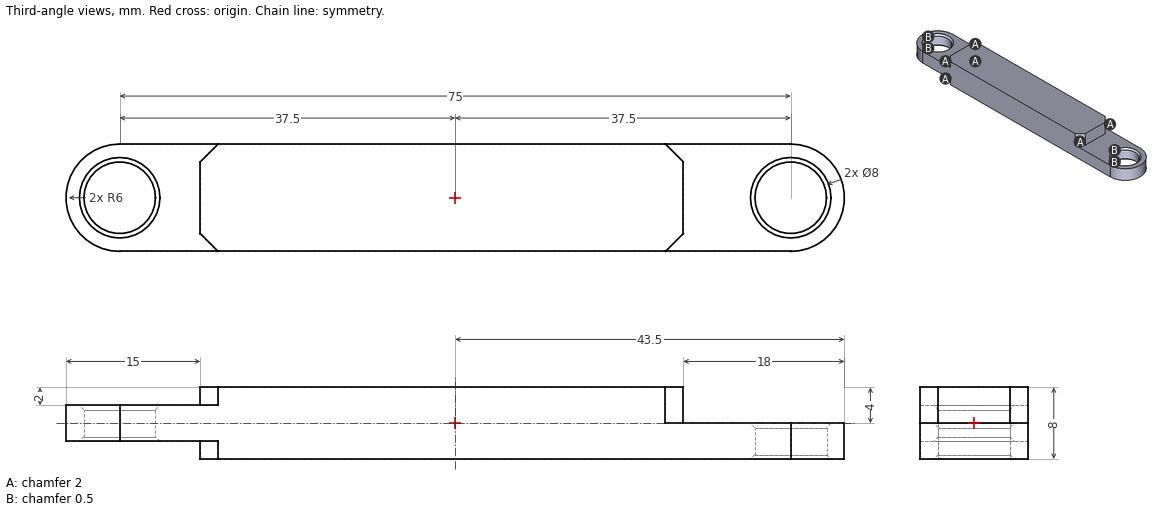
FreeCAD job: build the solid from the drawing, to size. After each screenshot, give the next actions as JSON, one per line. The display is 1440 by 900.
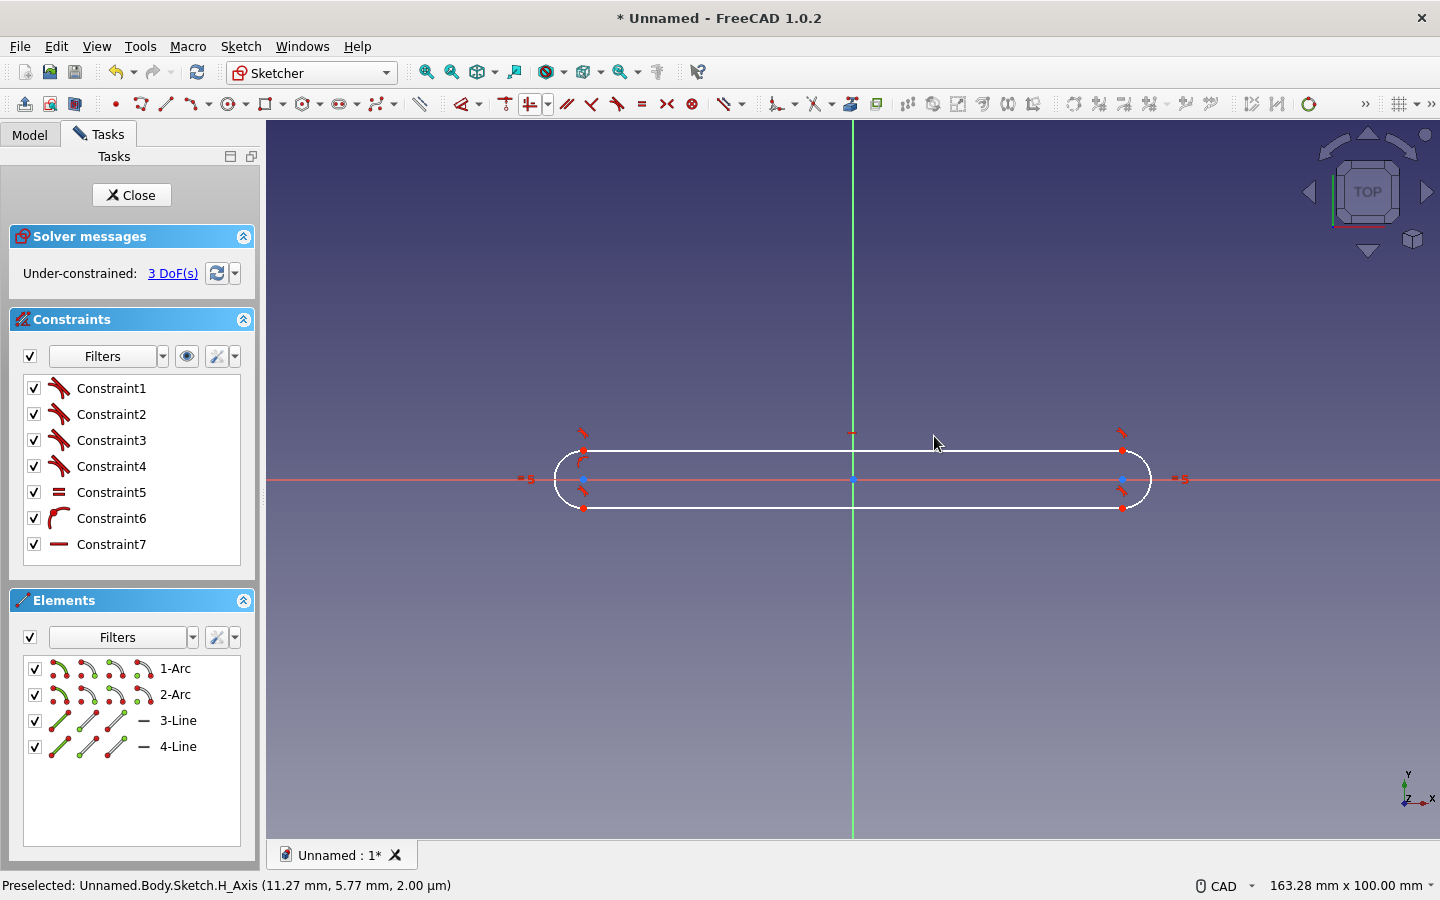
{"action": "left_click", "coordinate": [460, 104]}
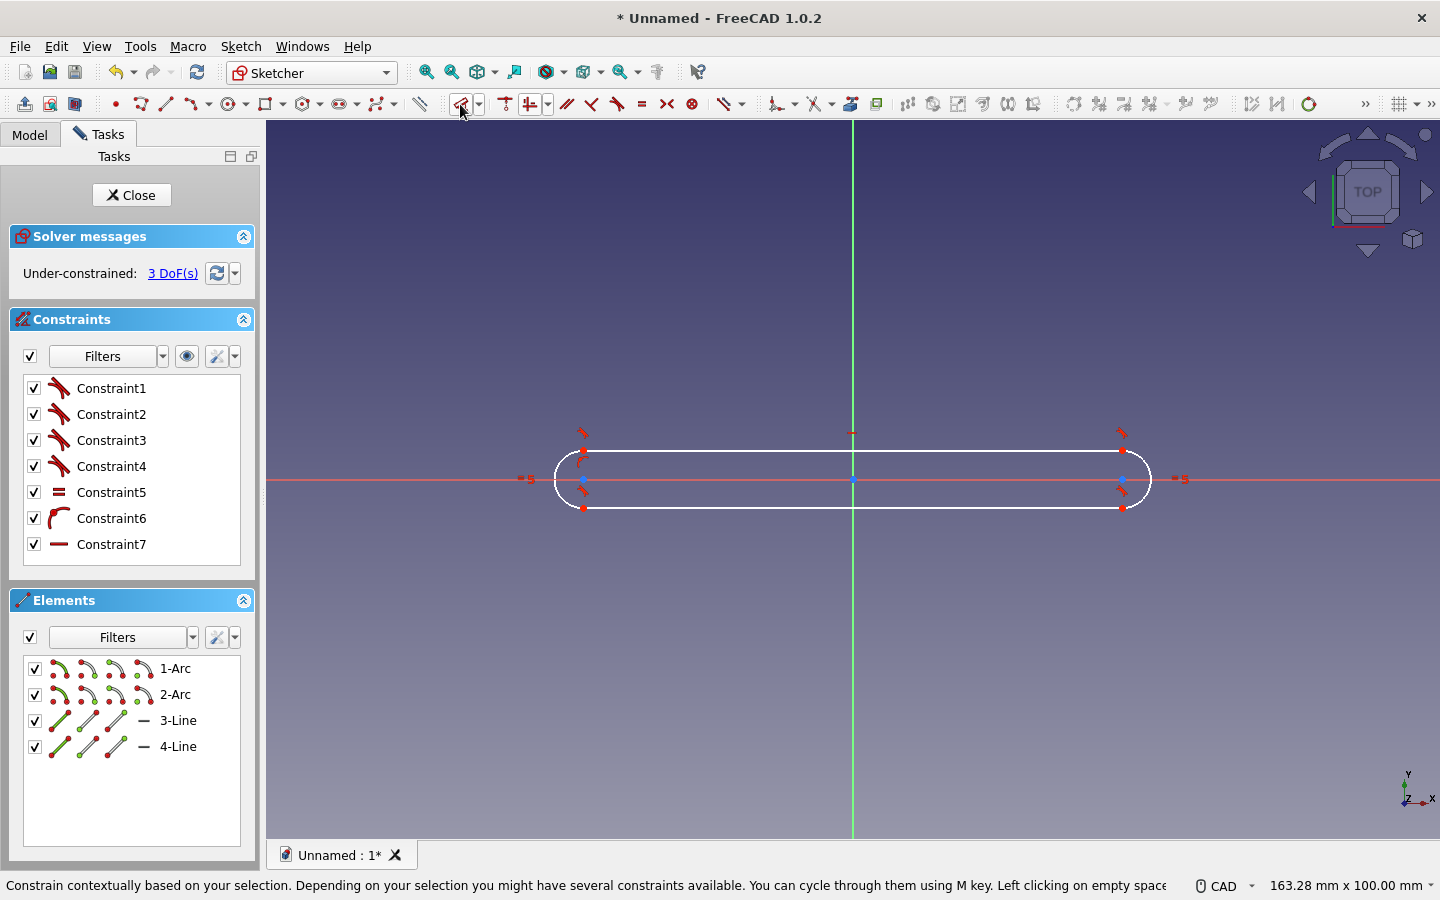
{"action": "left_click", "coordinate": [560, 463]}
{"action": "left_click", "coordinate": [534, 444]}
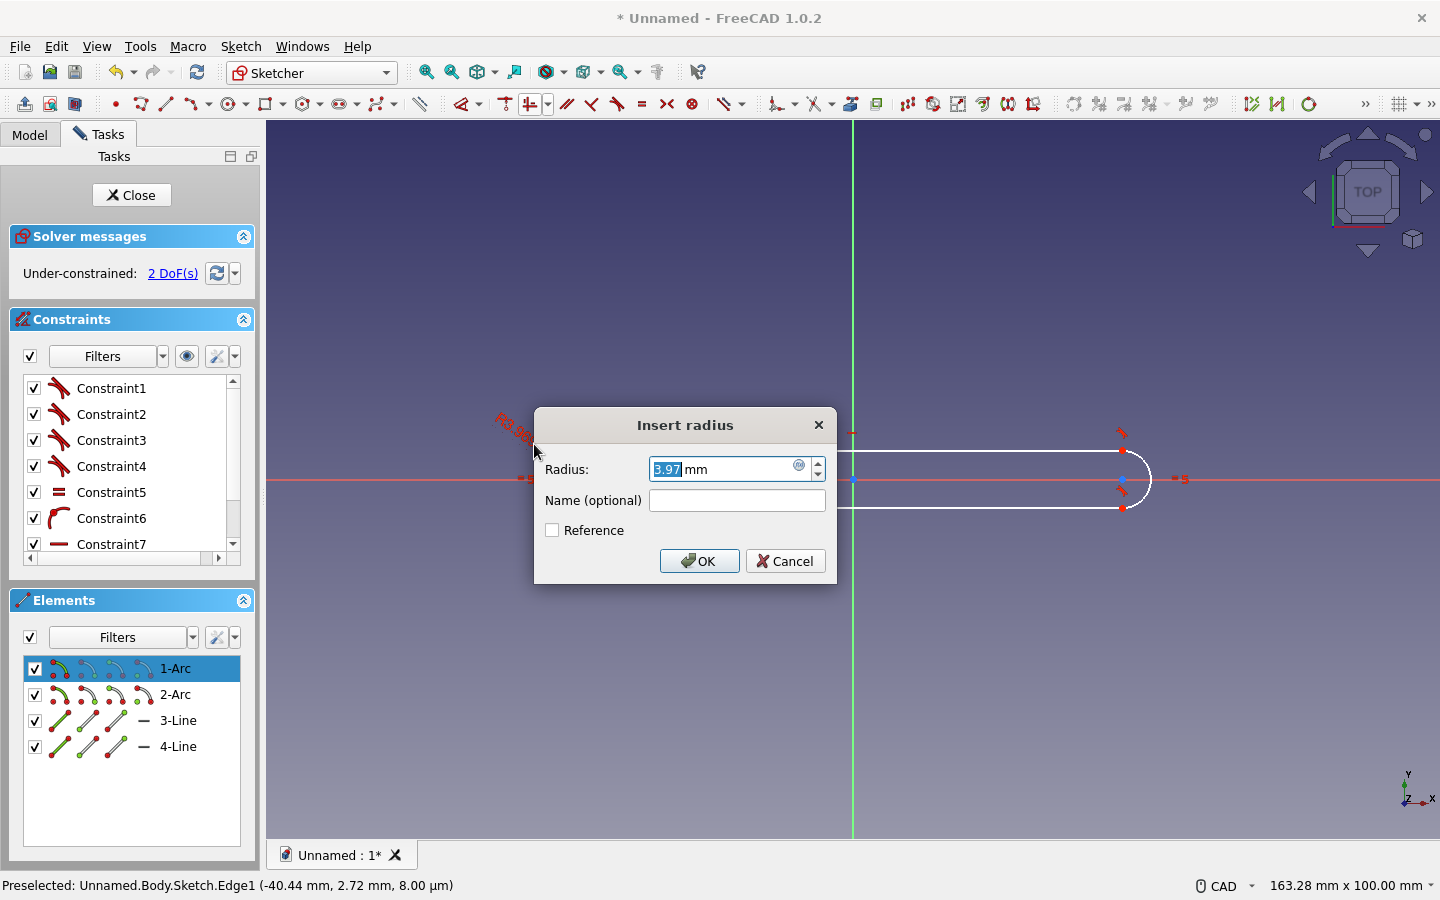
{"action": "type", "text": "6"}
{"action": "key", "text": "Return"}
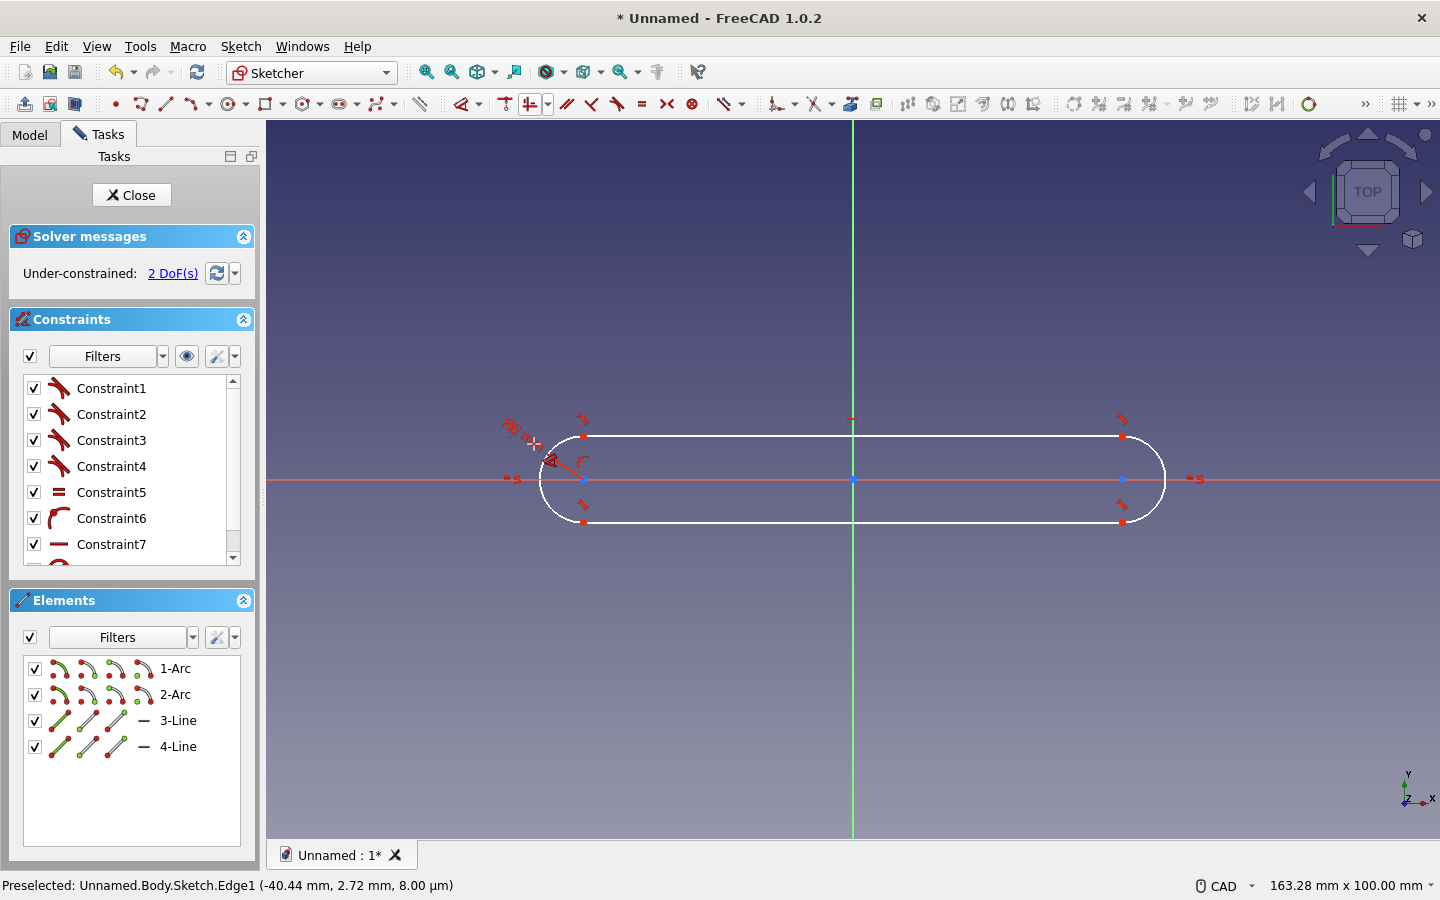
{"action": "left_click", "coordinate": [745, 436]}
{"action": "left_click", "coordinate": [729, 402]}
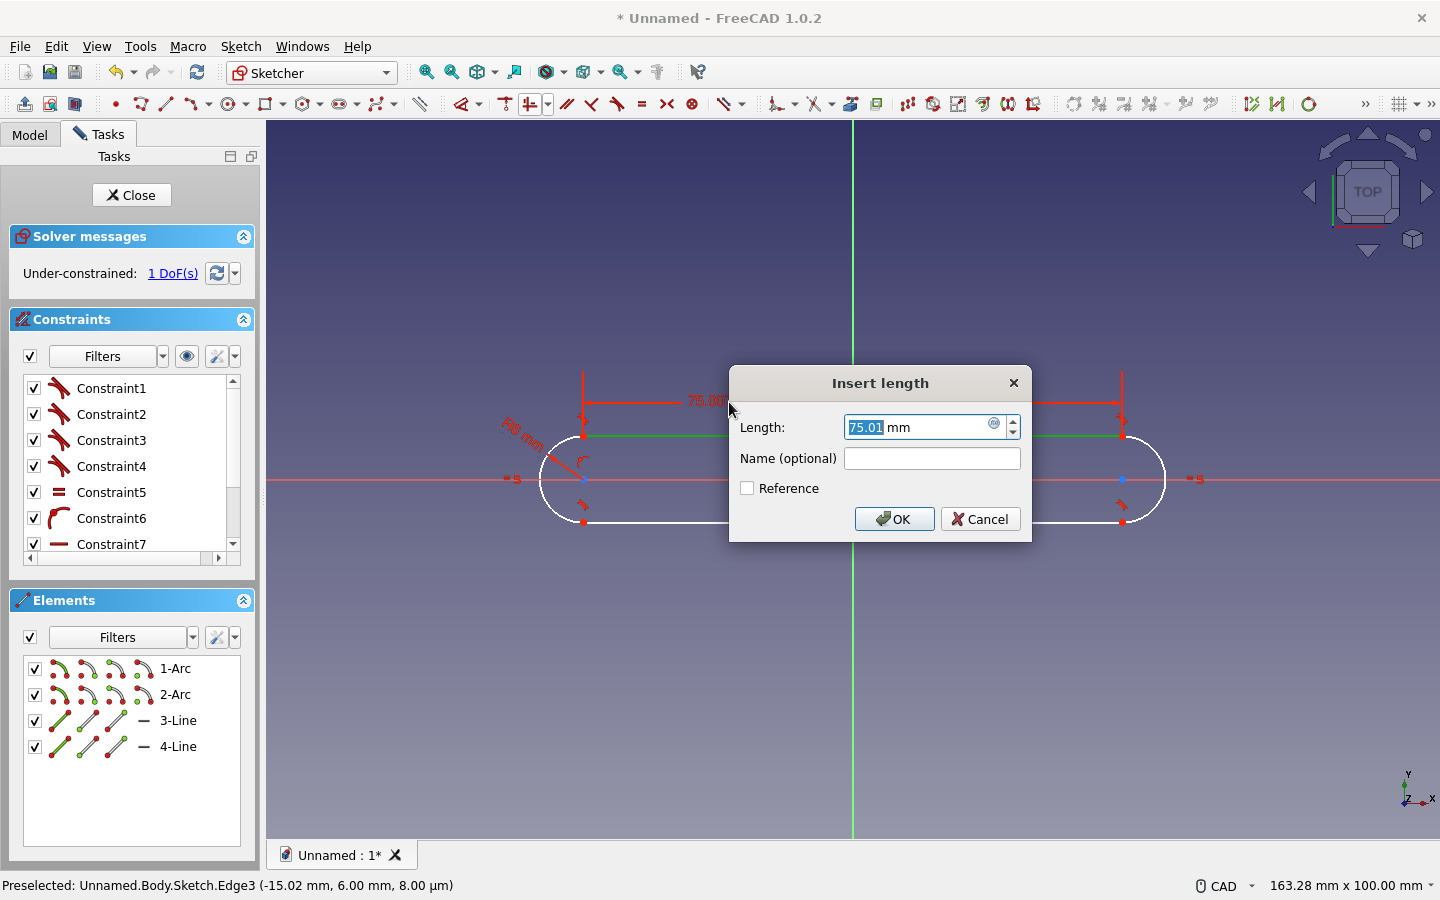
{"action": "type", "text": "75"}
{"action": "key", "text": "Return"}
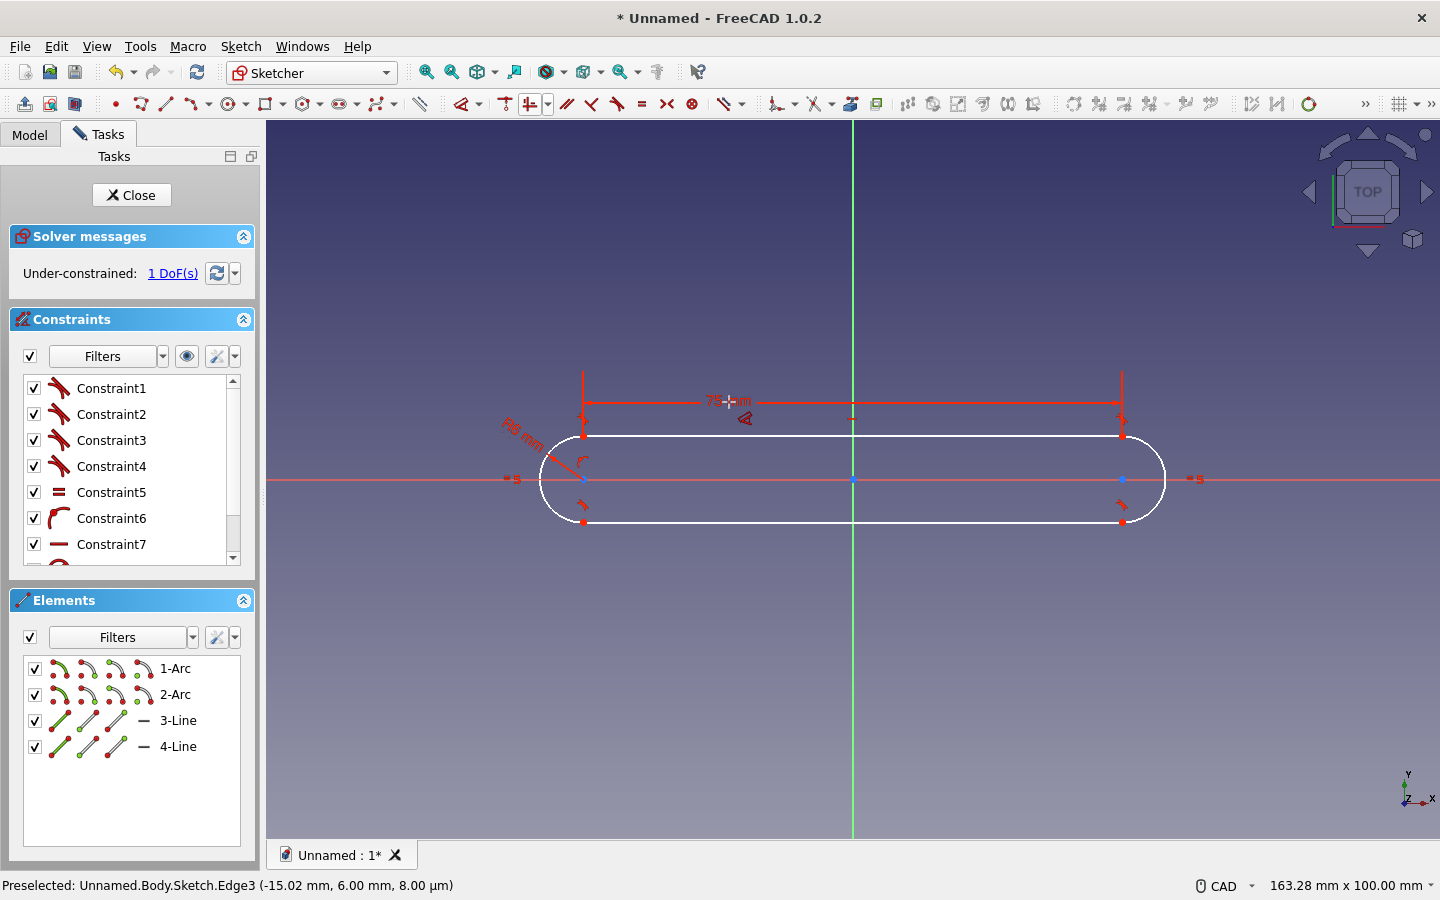
{"action": "left_click", "coordinate": [583, 436]}
{"action": "left_click", "coordinate": [656, 402]}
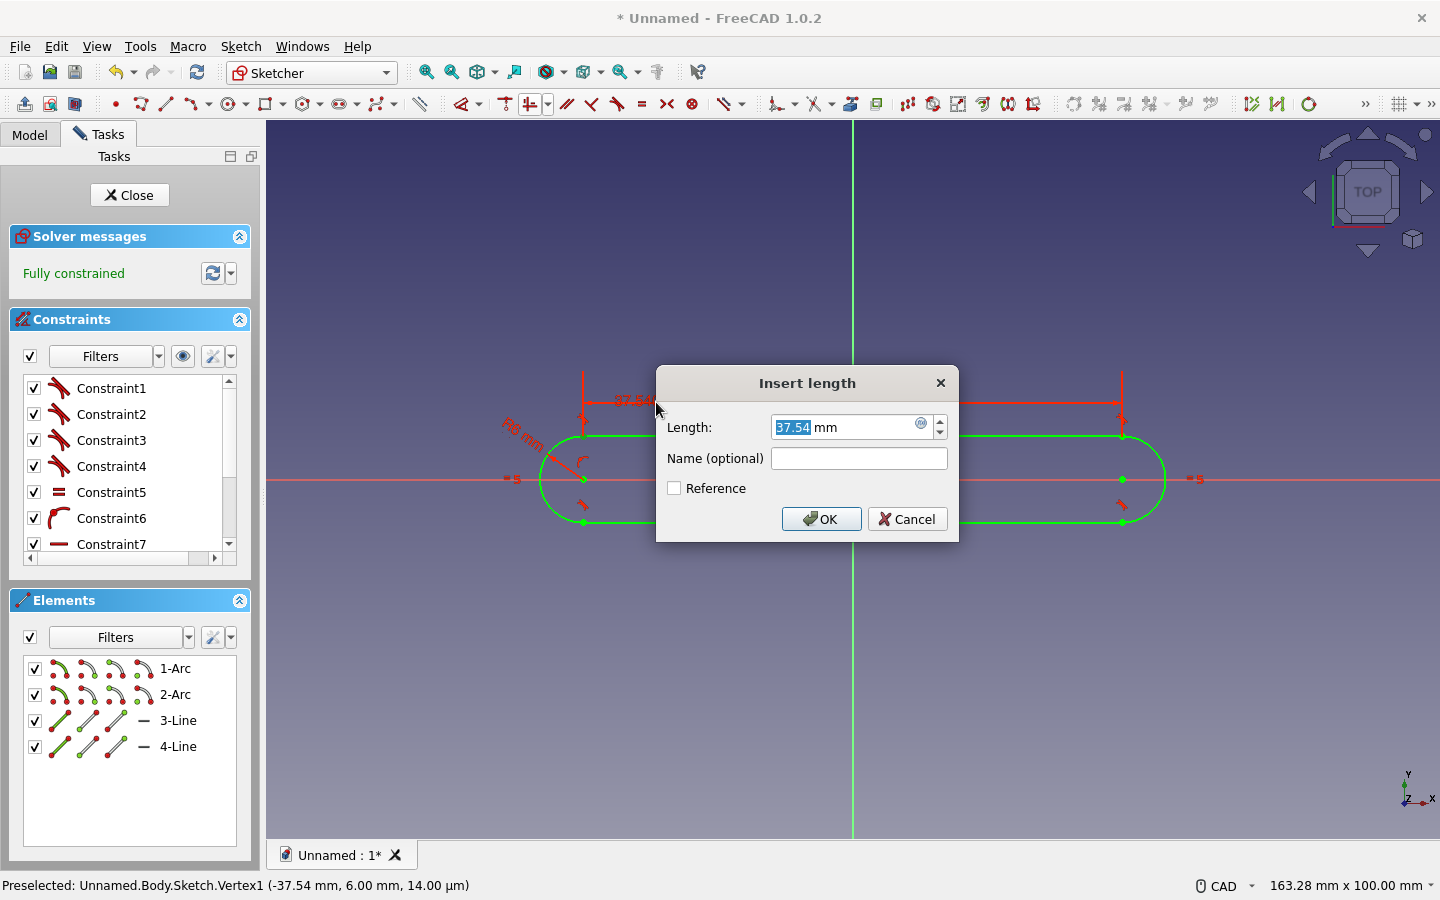
{"action": "type", "text": "37.5"}
{"action": "key", "text": "Return"}
{"action": "key", "text": "Escape"}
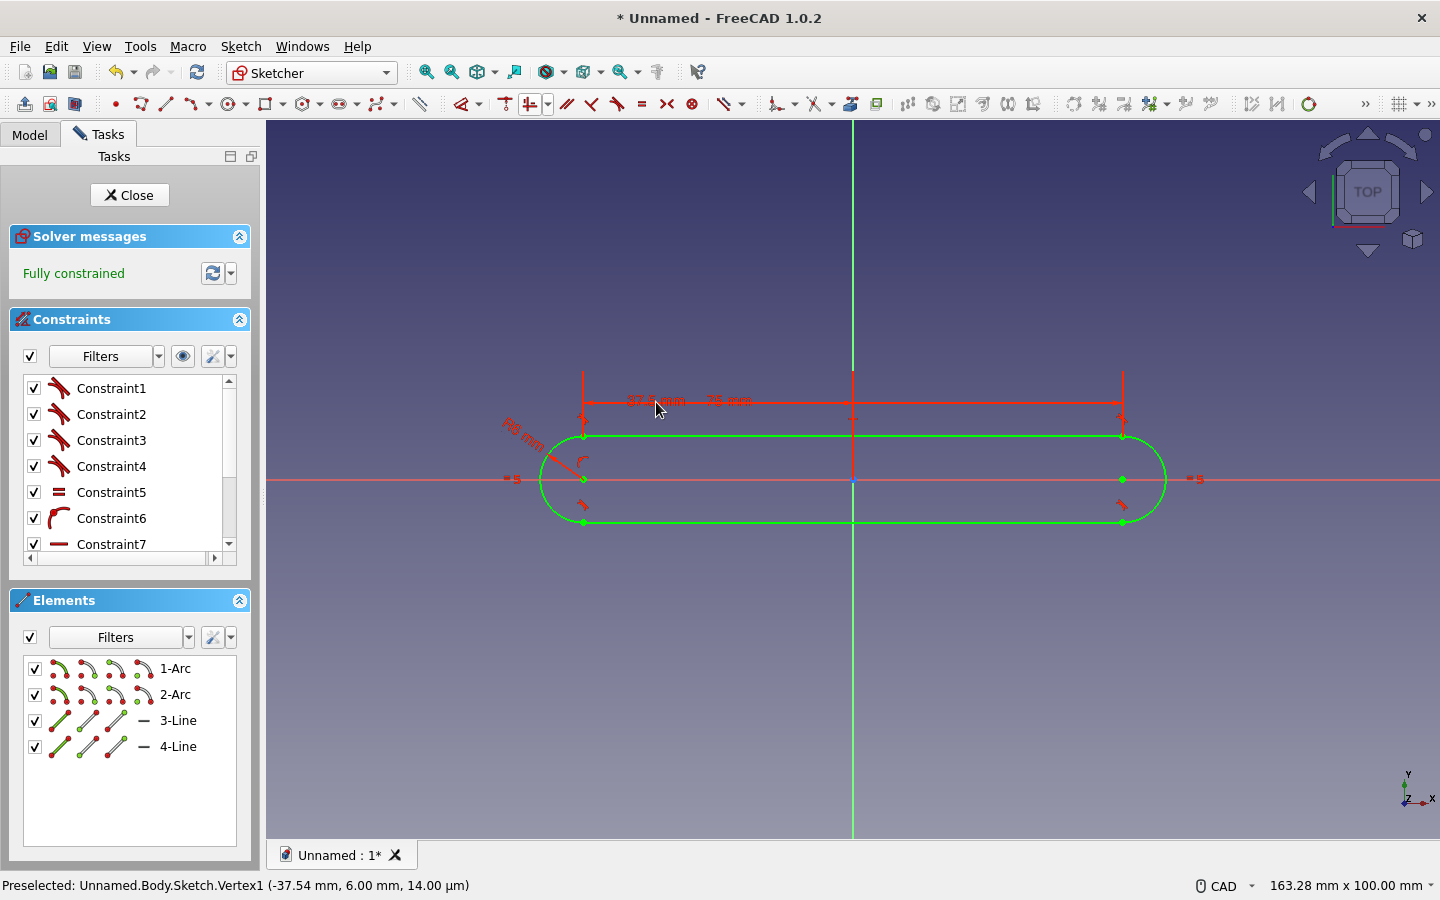
{"action": "left_click", "coordinate": [130, 195]}